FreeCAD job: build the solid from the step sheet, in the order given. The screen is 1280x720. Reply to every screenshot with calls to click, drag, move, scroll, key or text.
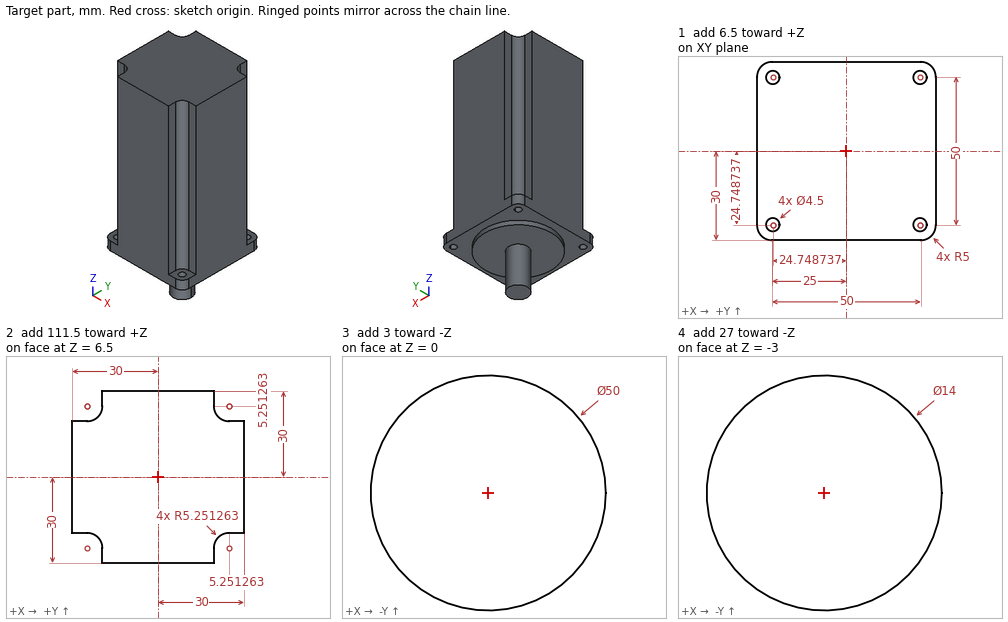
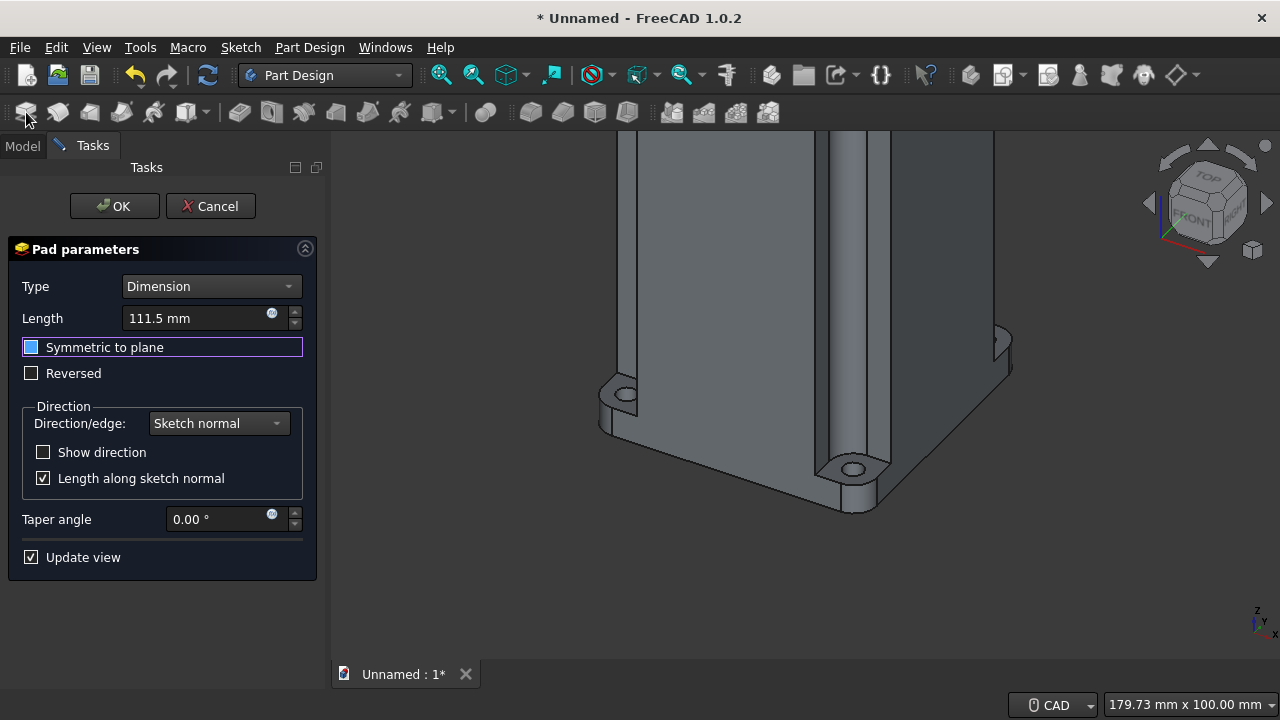
click(115, 206)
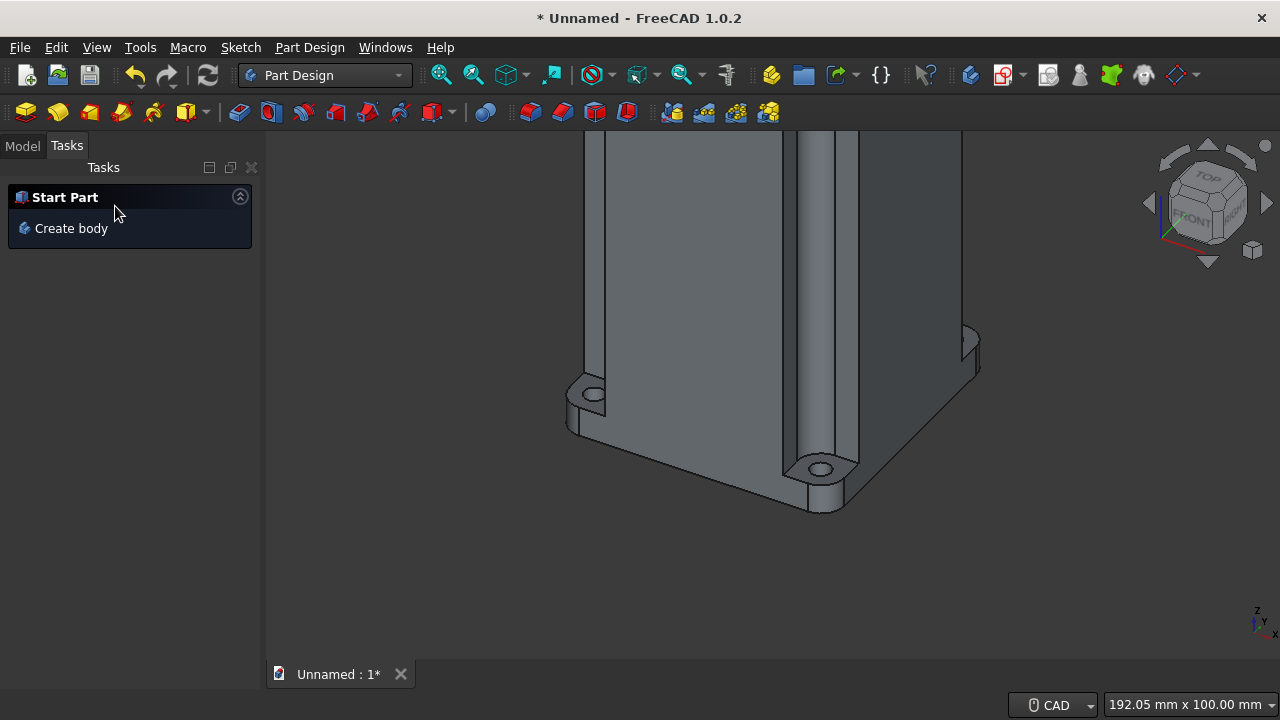
click(442, 76)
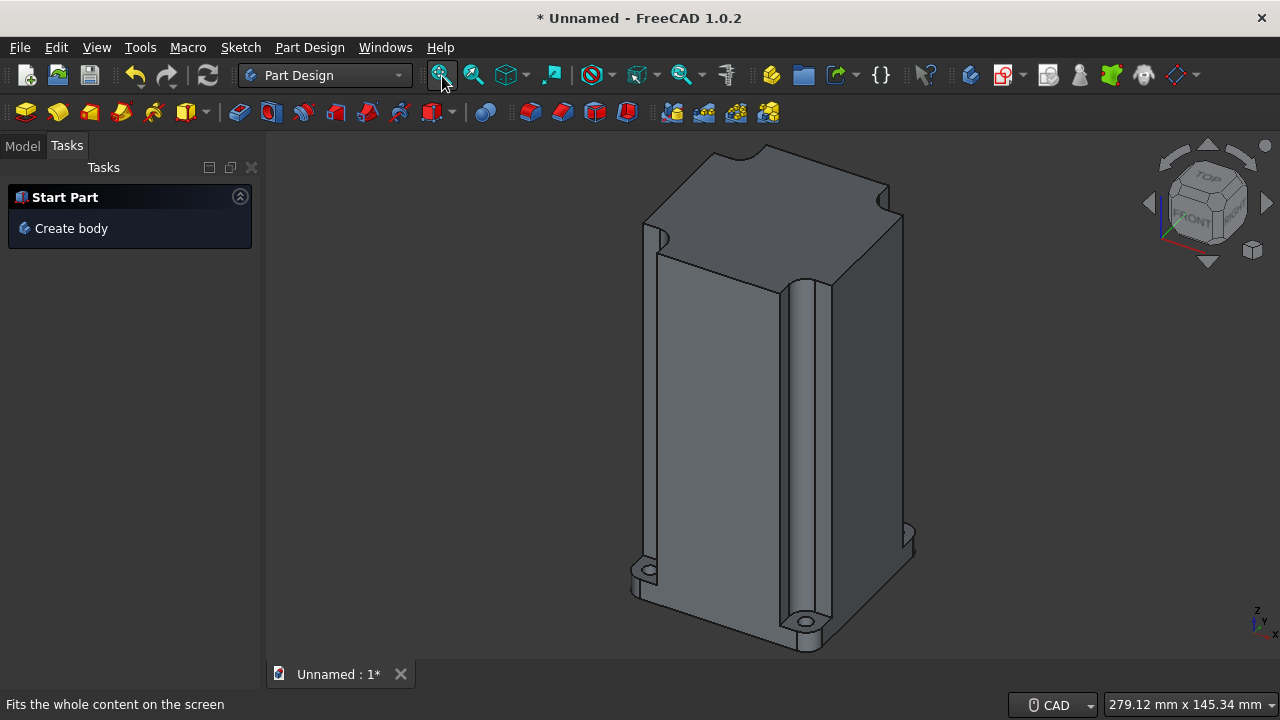
key(5)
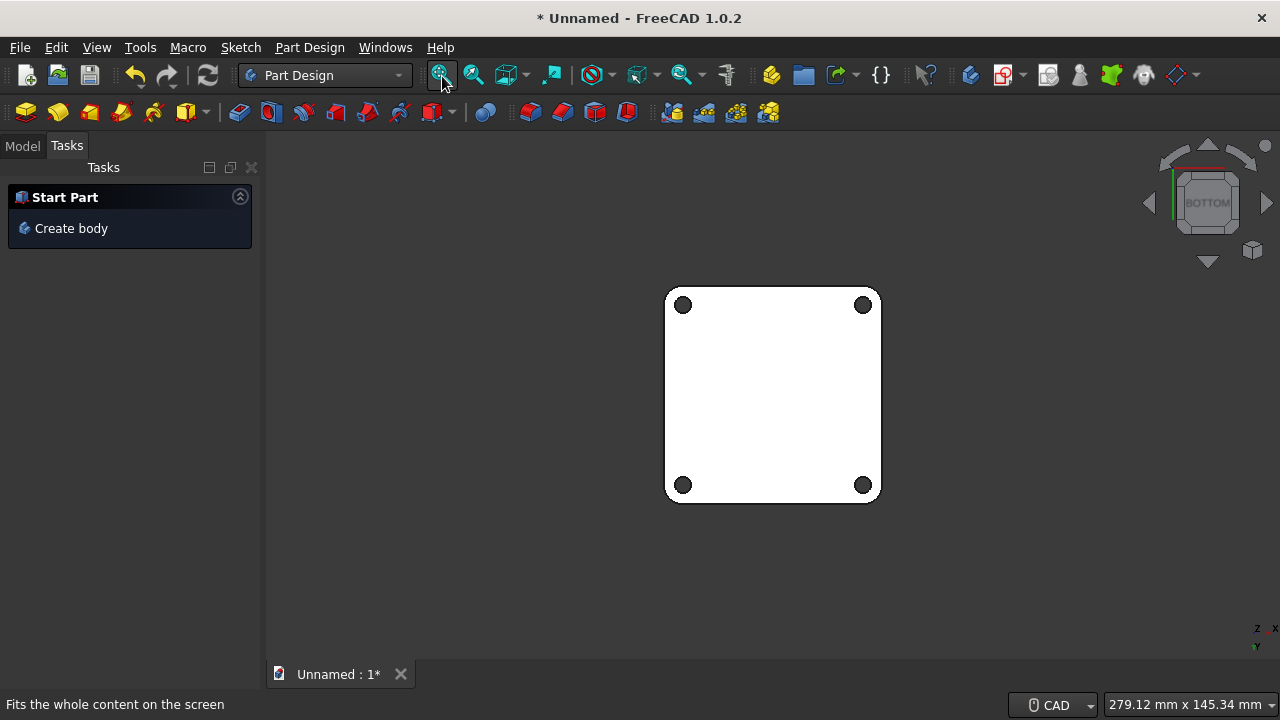
click(442, 76)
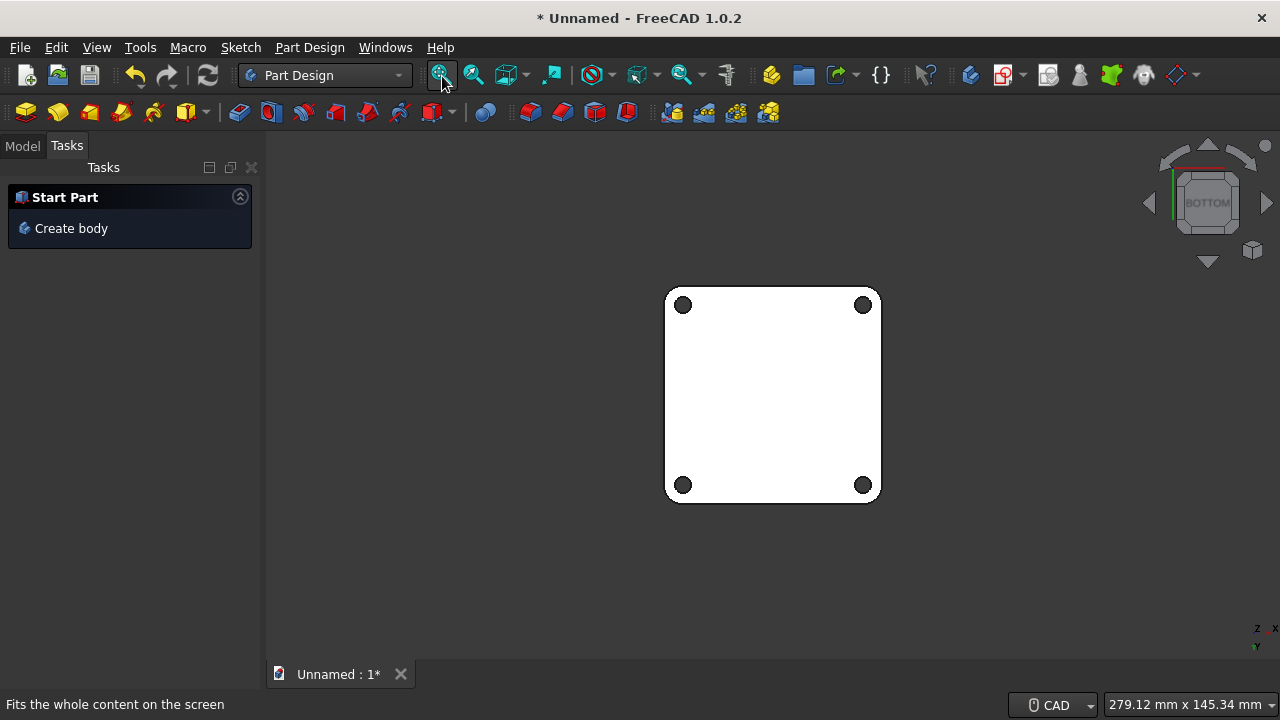
click(773, 394)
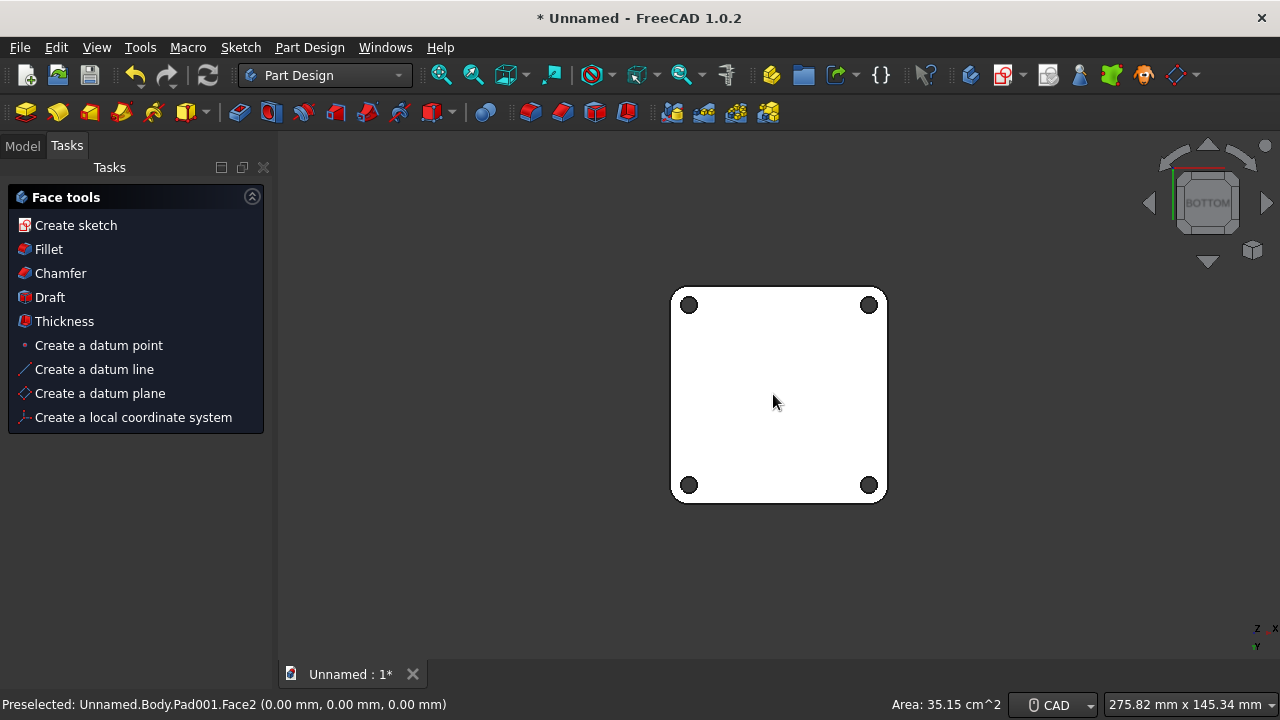
click(1004, 76)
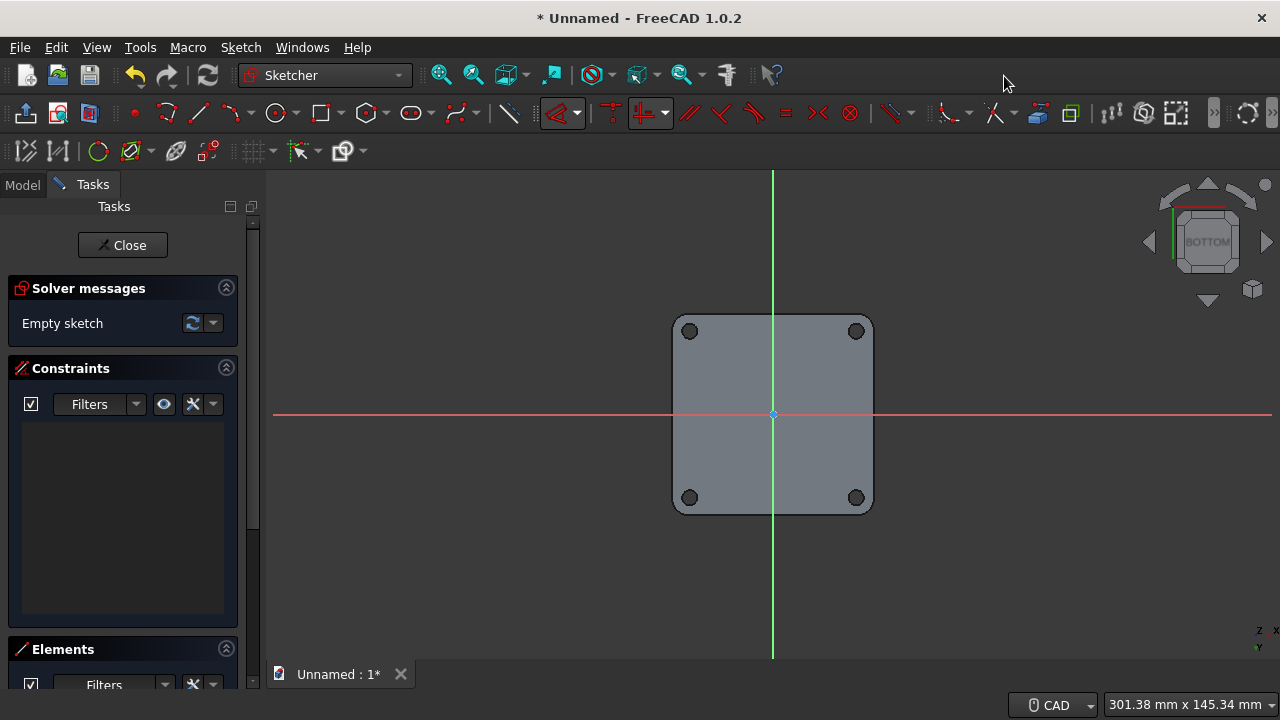
scroll(856, 415, up, 3)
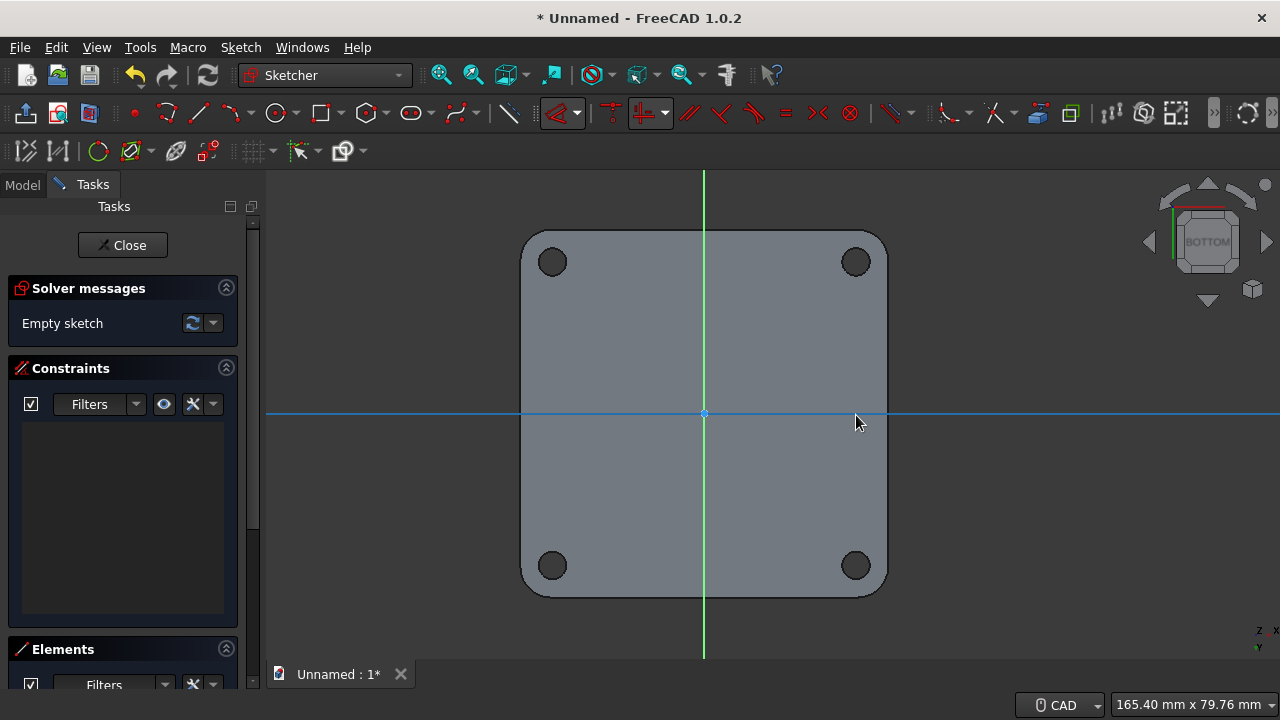
click(276, 114)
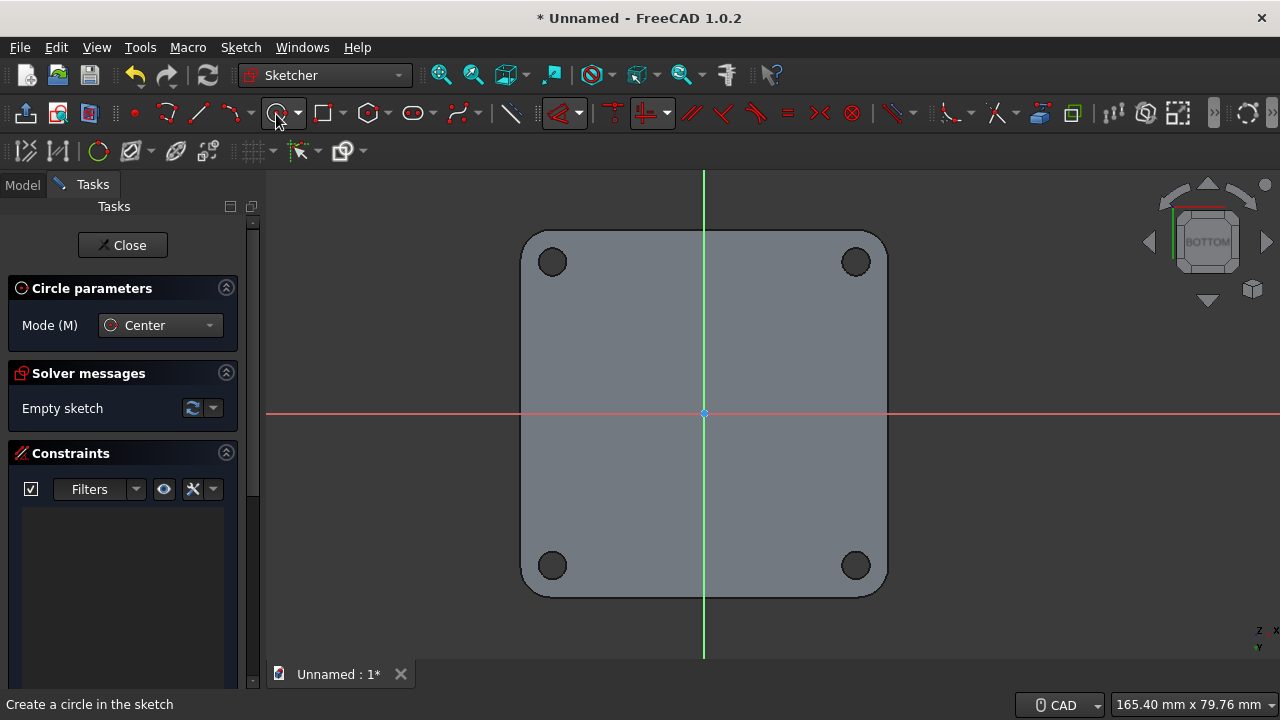
click(704, 414)
click(813, 305)
key(Escape)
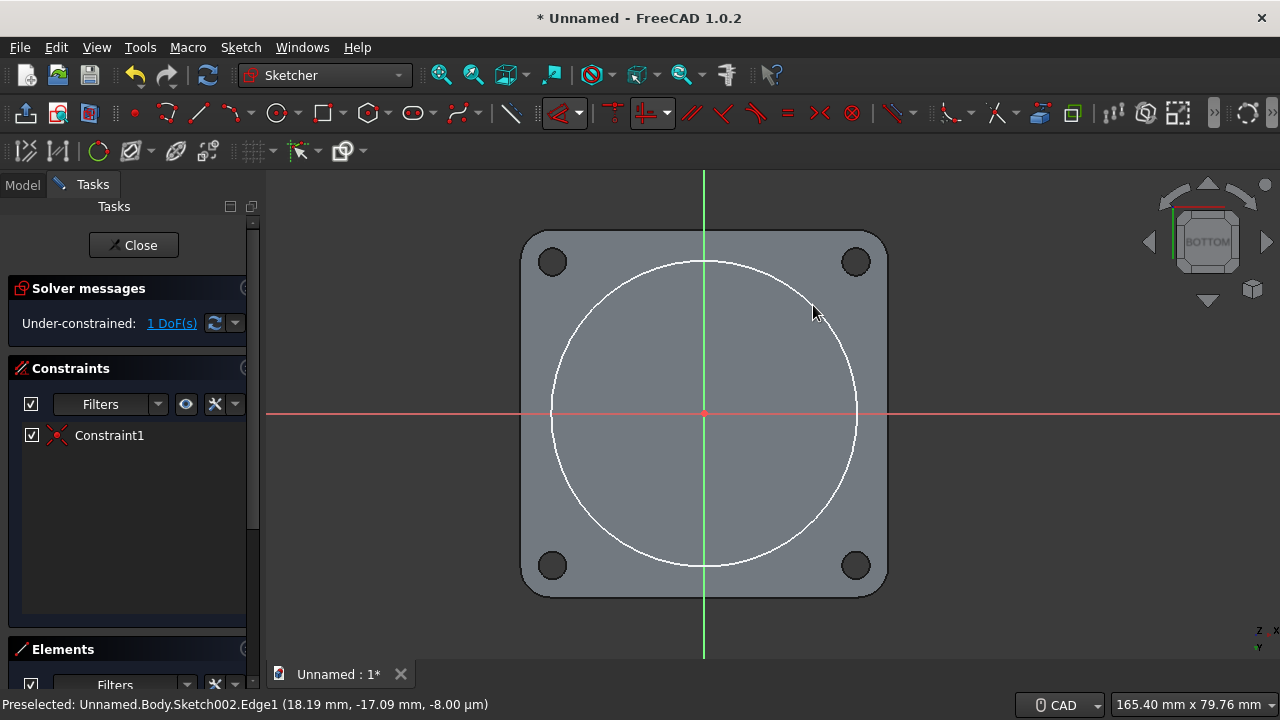
click(812, 305)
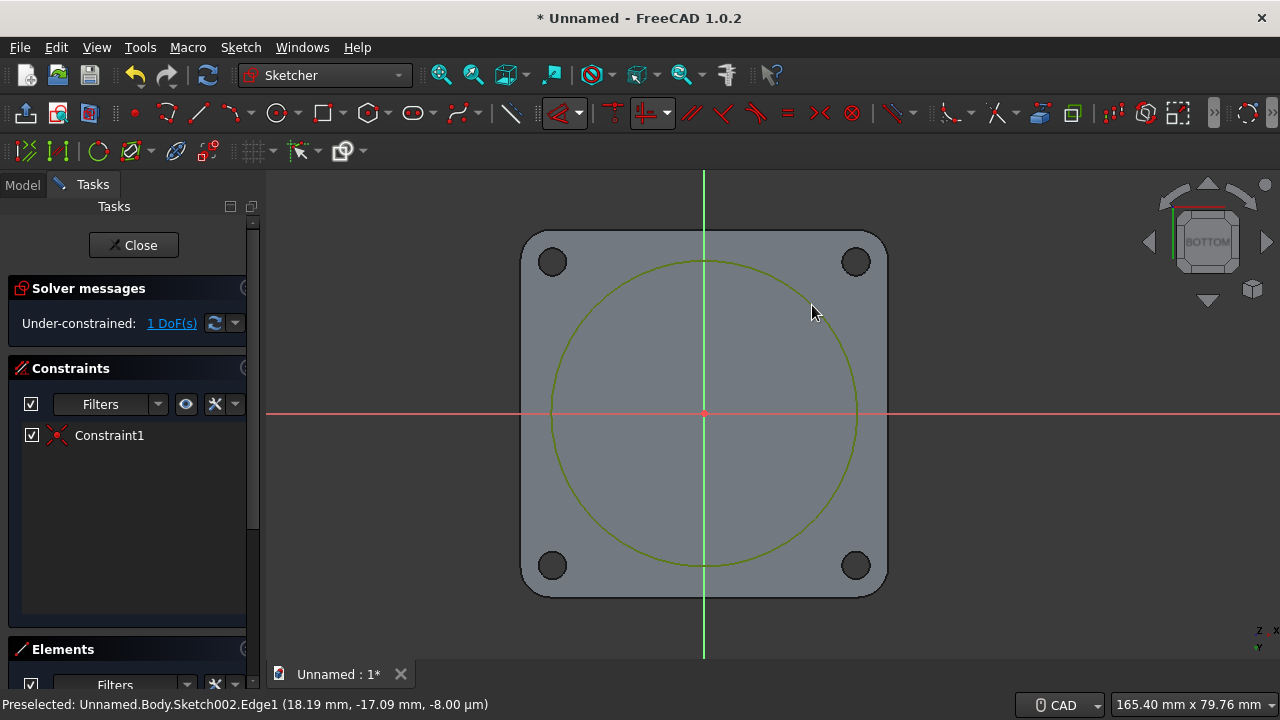
key(k)
key(o)